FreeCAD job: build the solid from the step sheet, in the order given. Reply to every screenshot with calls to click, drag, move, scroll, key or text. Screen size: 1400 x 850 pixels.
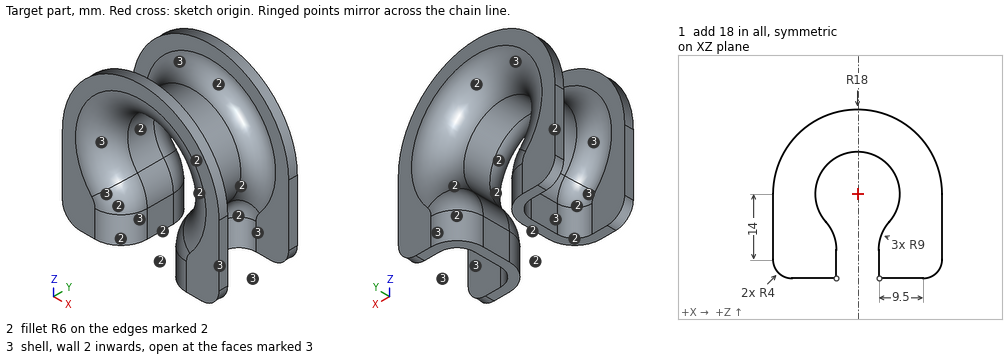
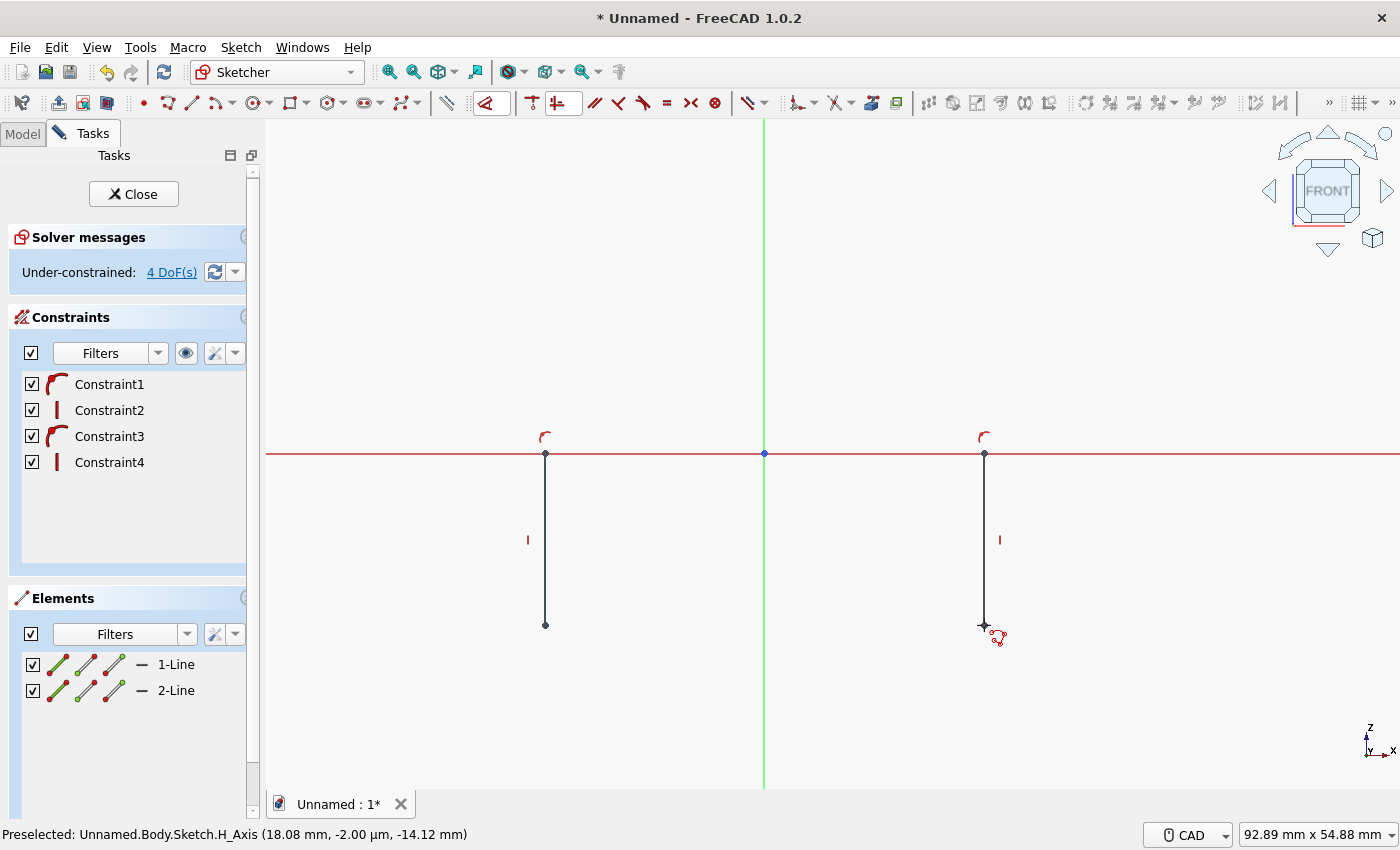
click(935, 673)
click(819, 673)
click(819, 599)
right_click(819, 599)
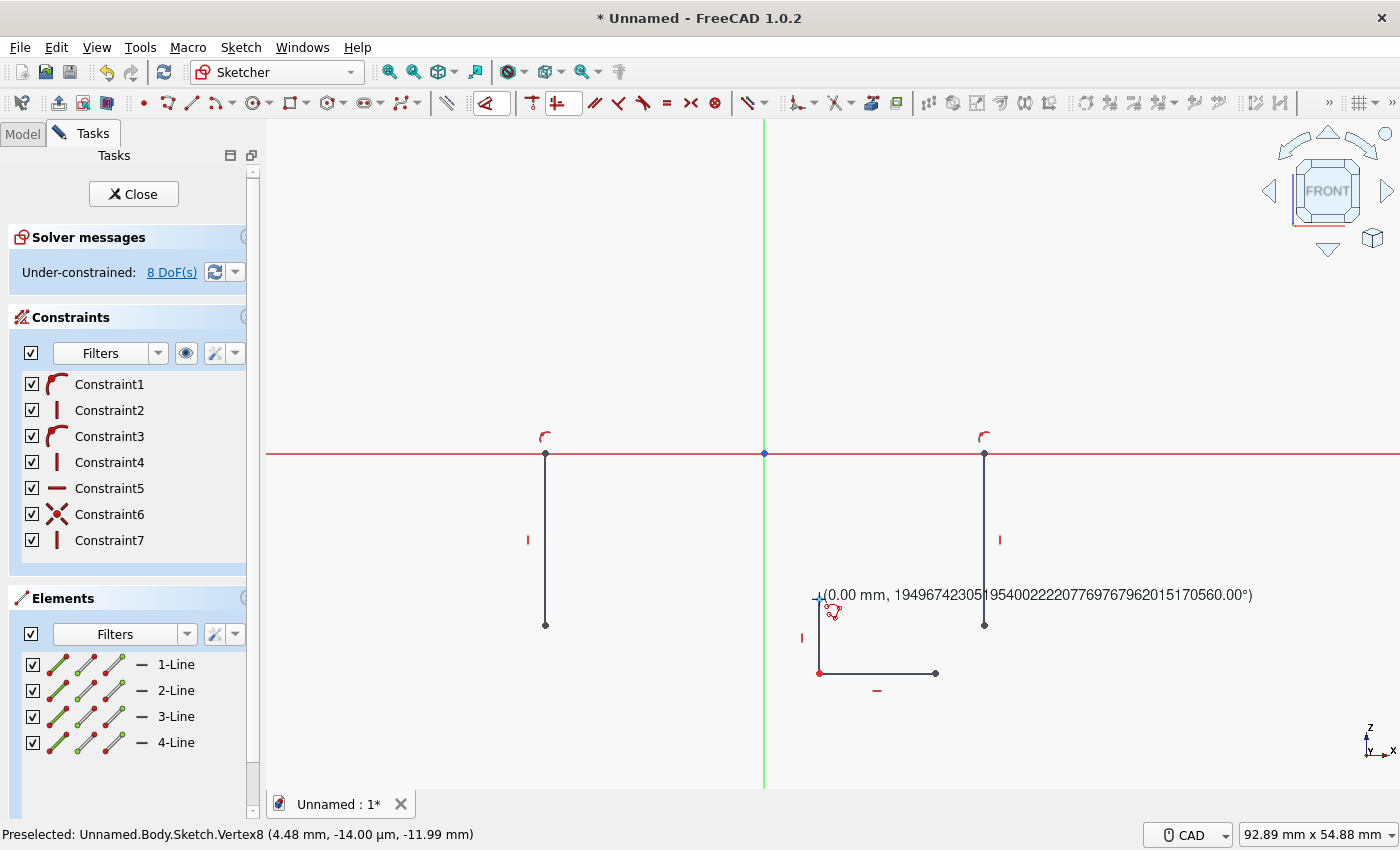
click(709, 599)
click(709, 673)
click(593, 673)
right_click(593, 673)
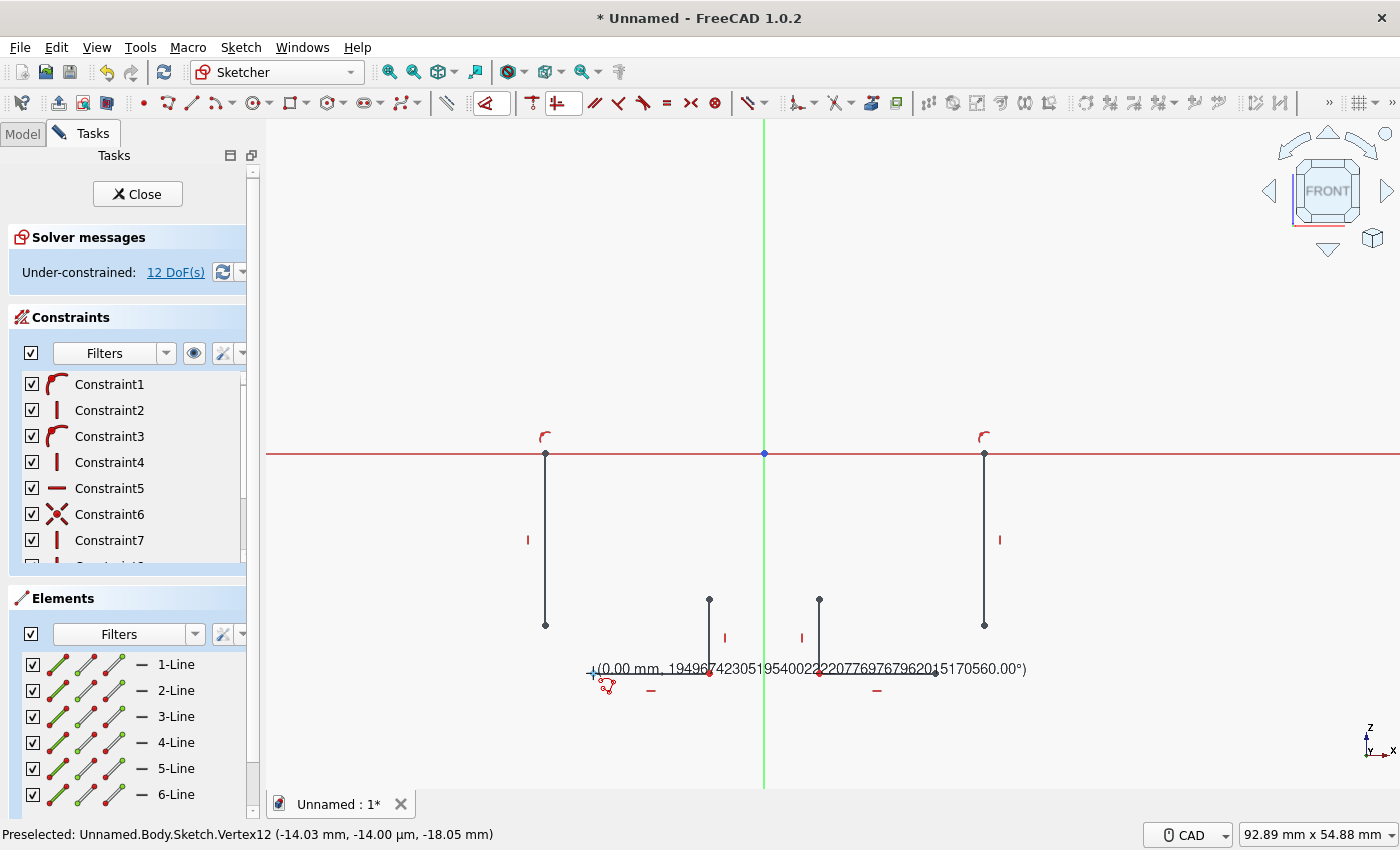
key(g)
key(3)
key(a)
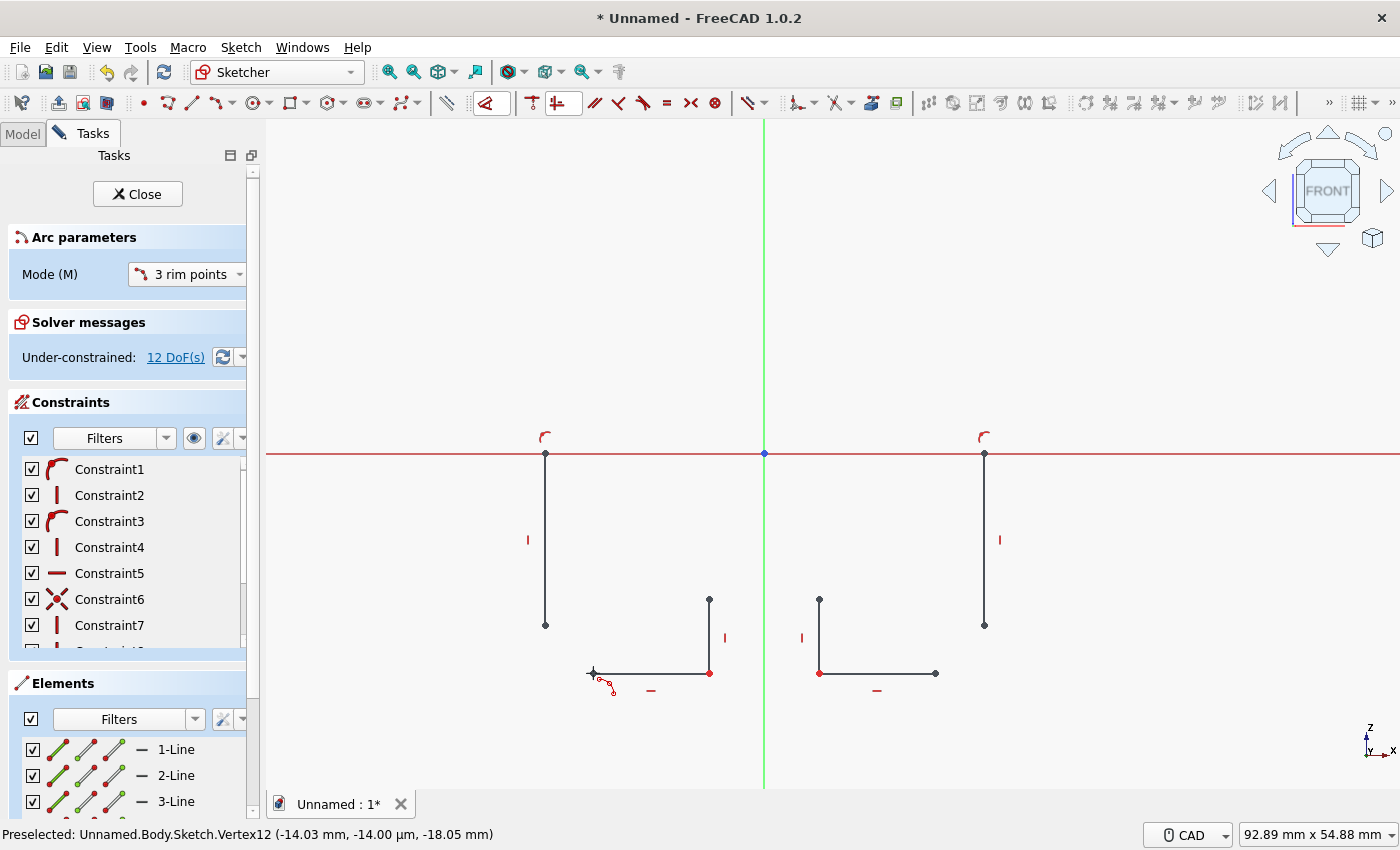
click(545, 454)
click(984, 454)
click(832, 245)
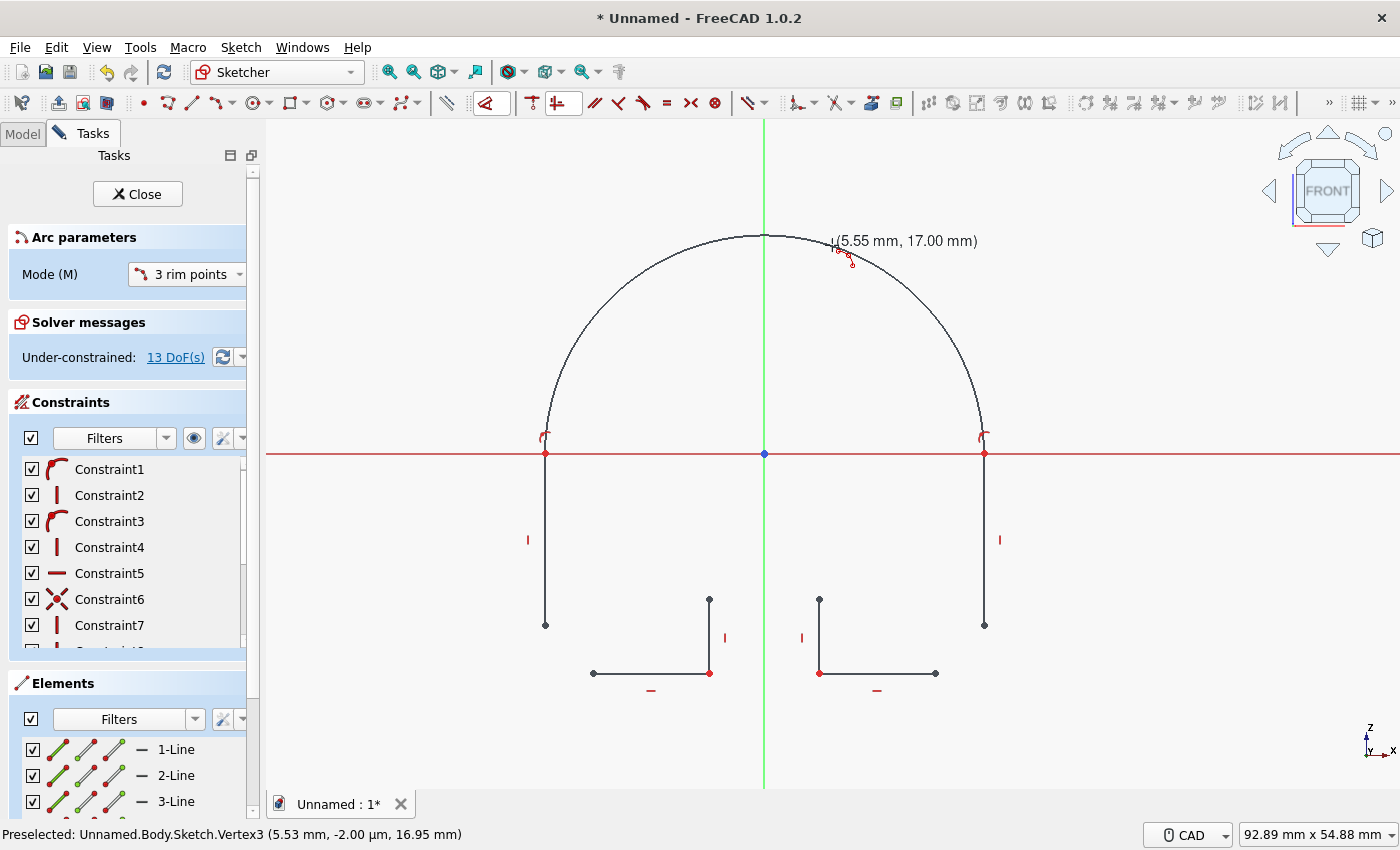
click(984, 626)
click(935, 674)
click(970, 659)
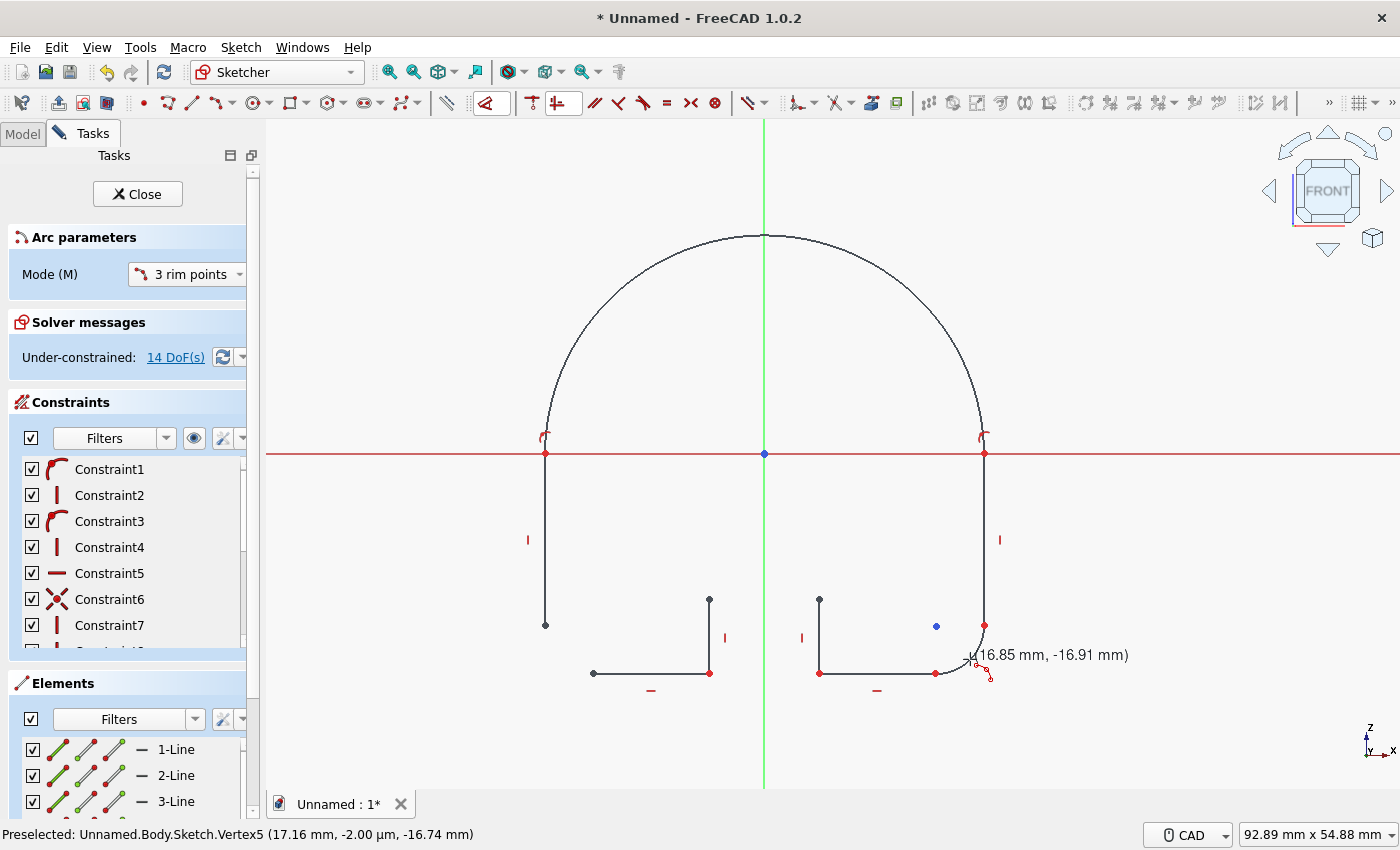
click(819, 600)
click(847, 526)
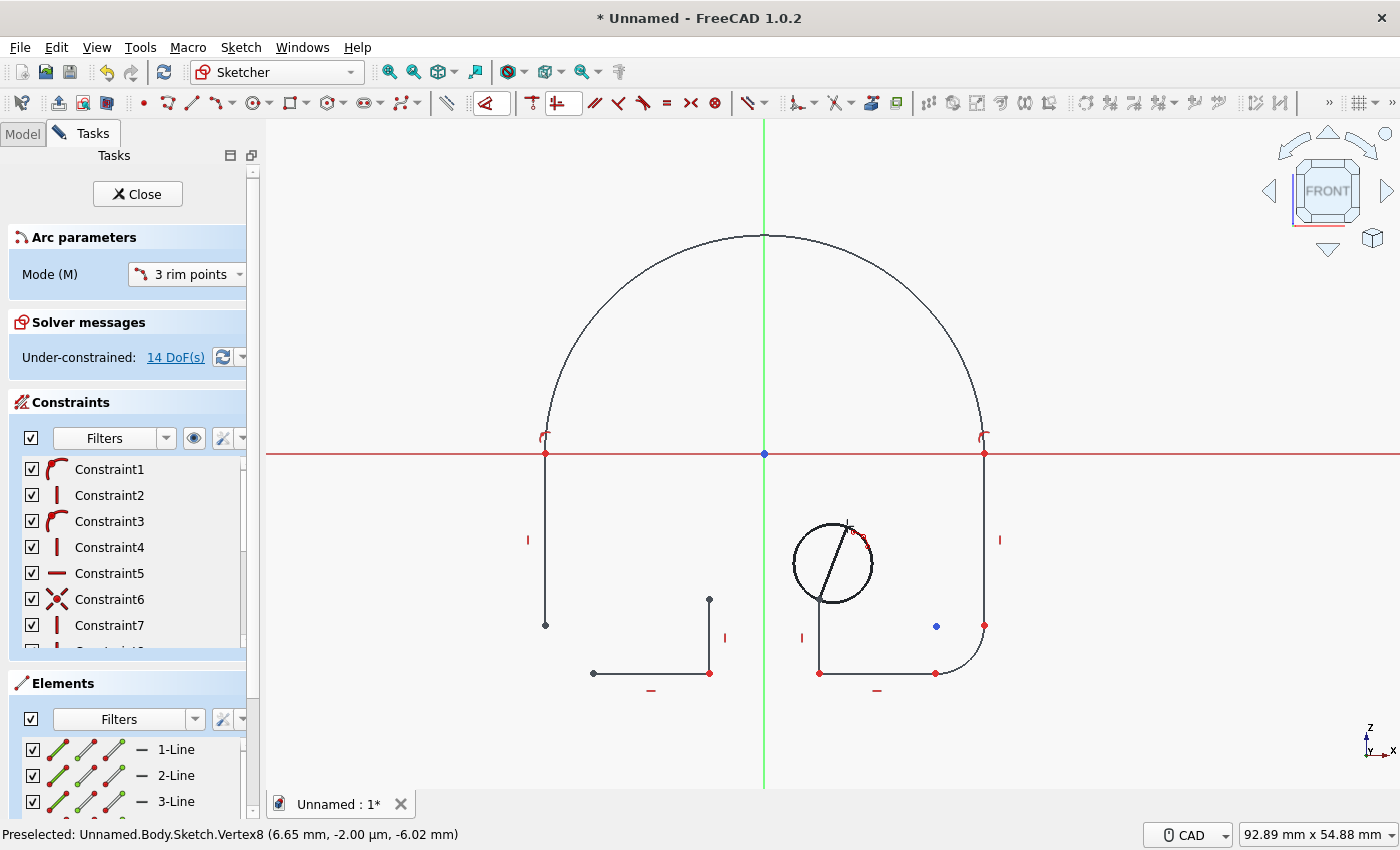
scroll(826, 560, up, 5)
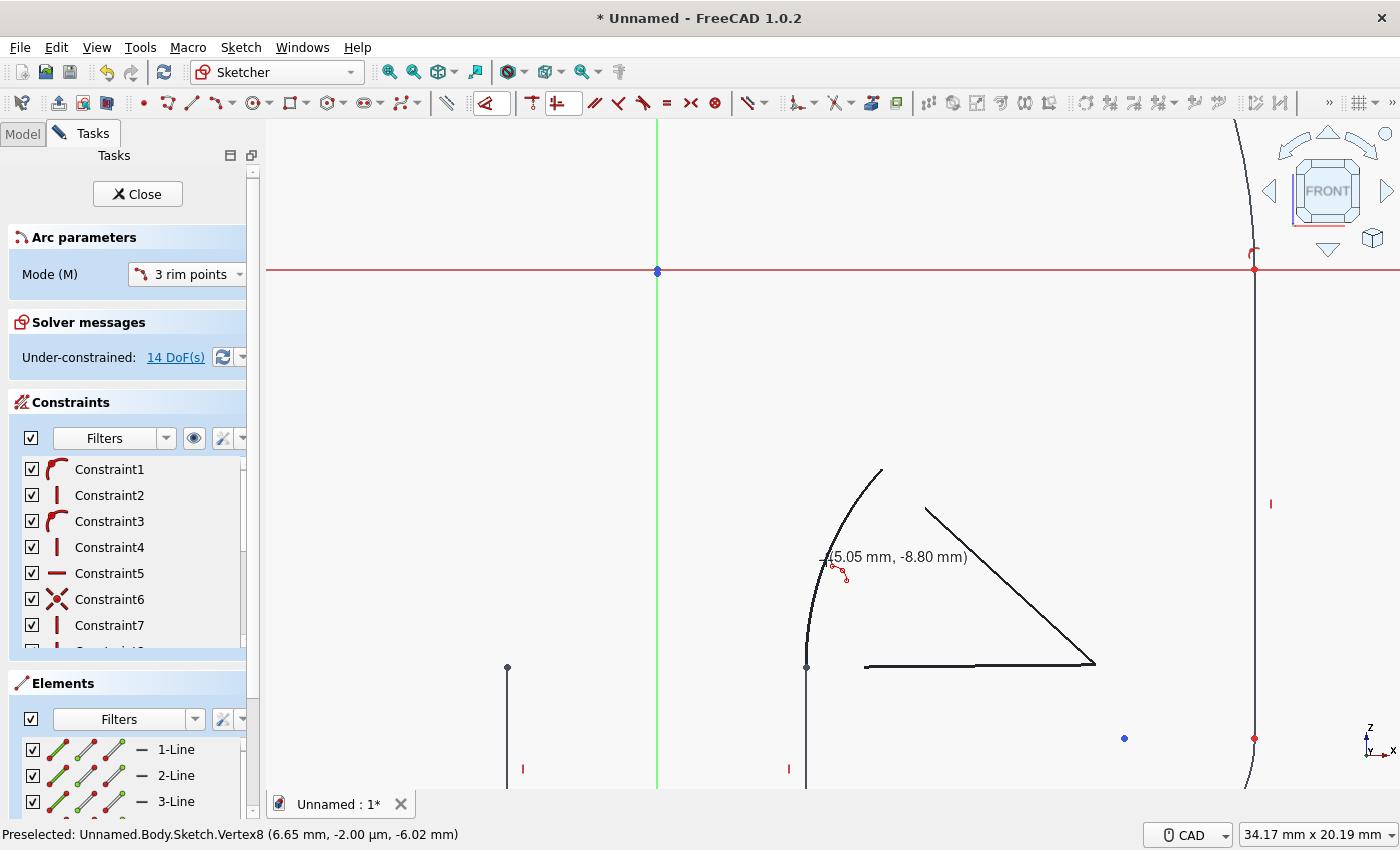
click(826, 559)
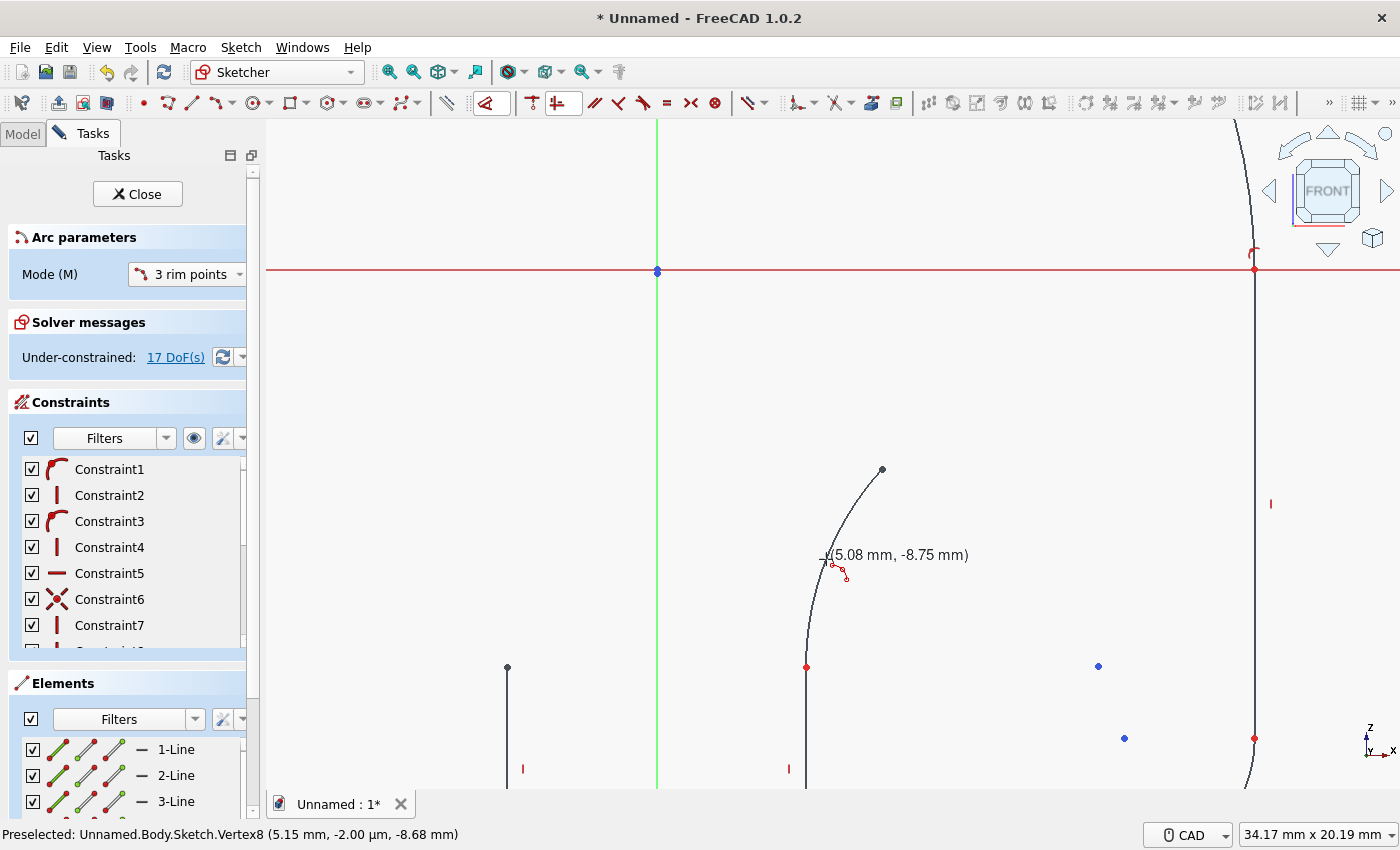
click(882, 469)
click(433, 467)